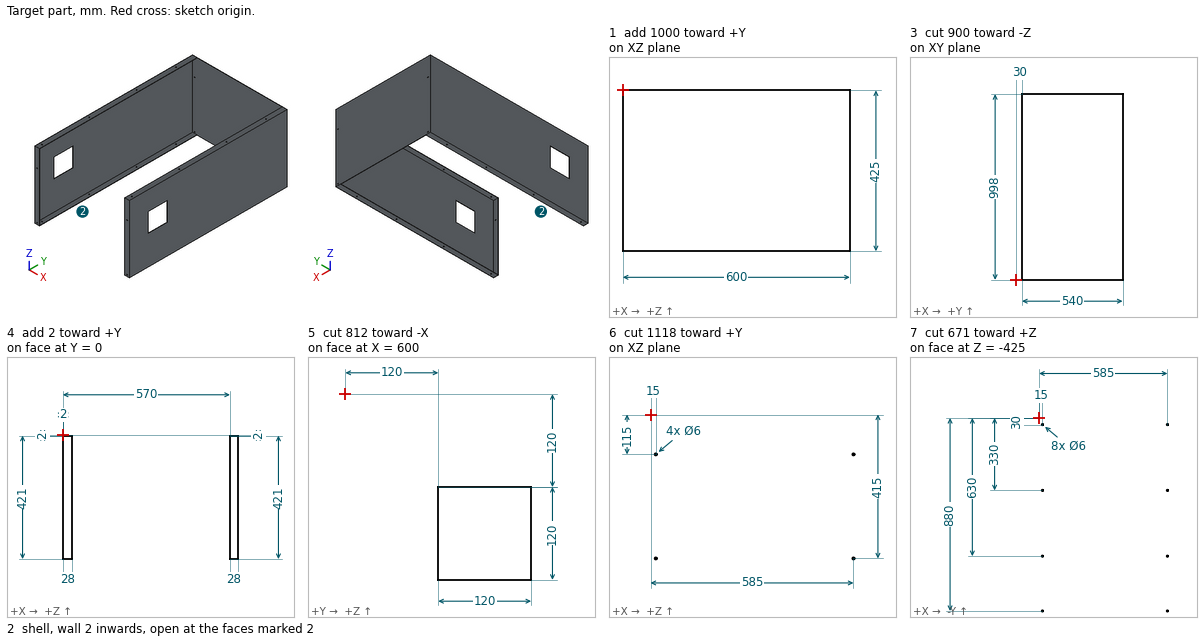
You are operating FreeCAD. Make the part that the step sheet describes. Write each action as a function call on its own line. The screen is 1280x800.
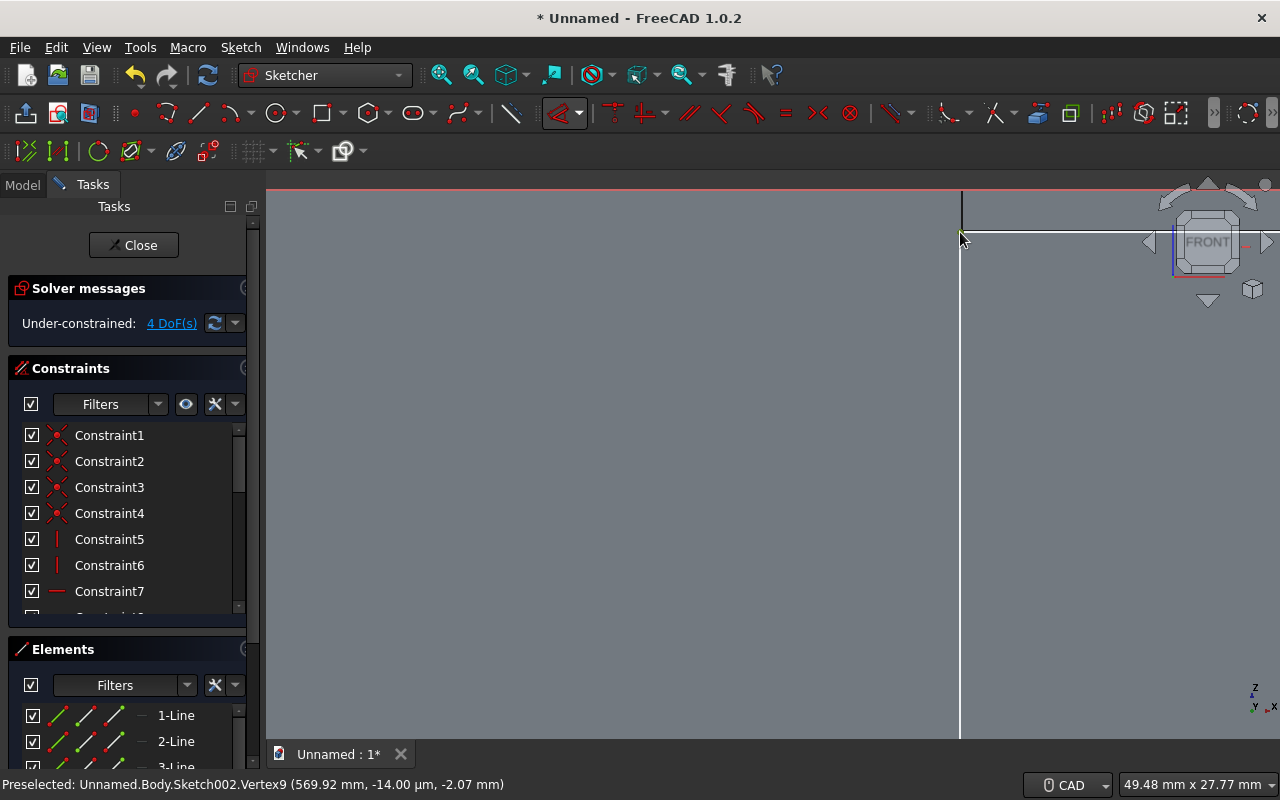
key(i)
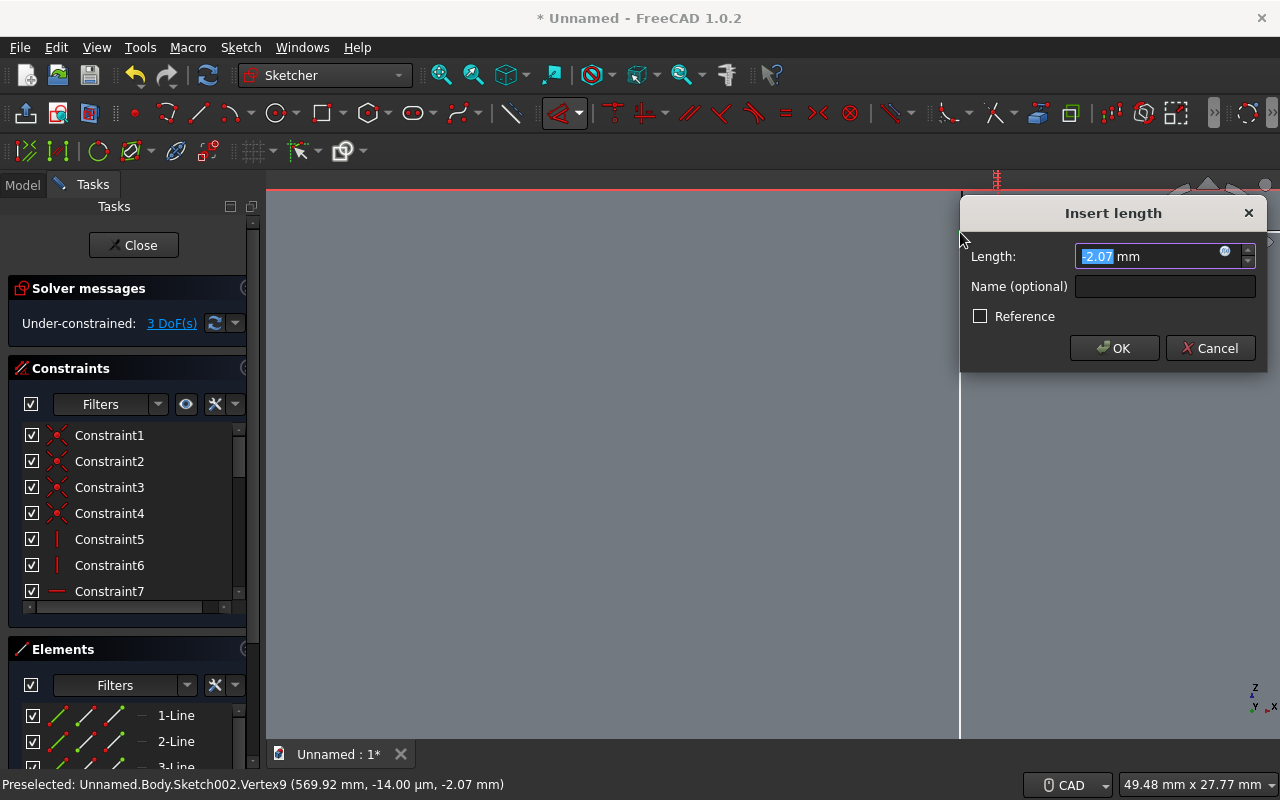
text(-2)
key(Return)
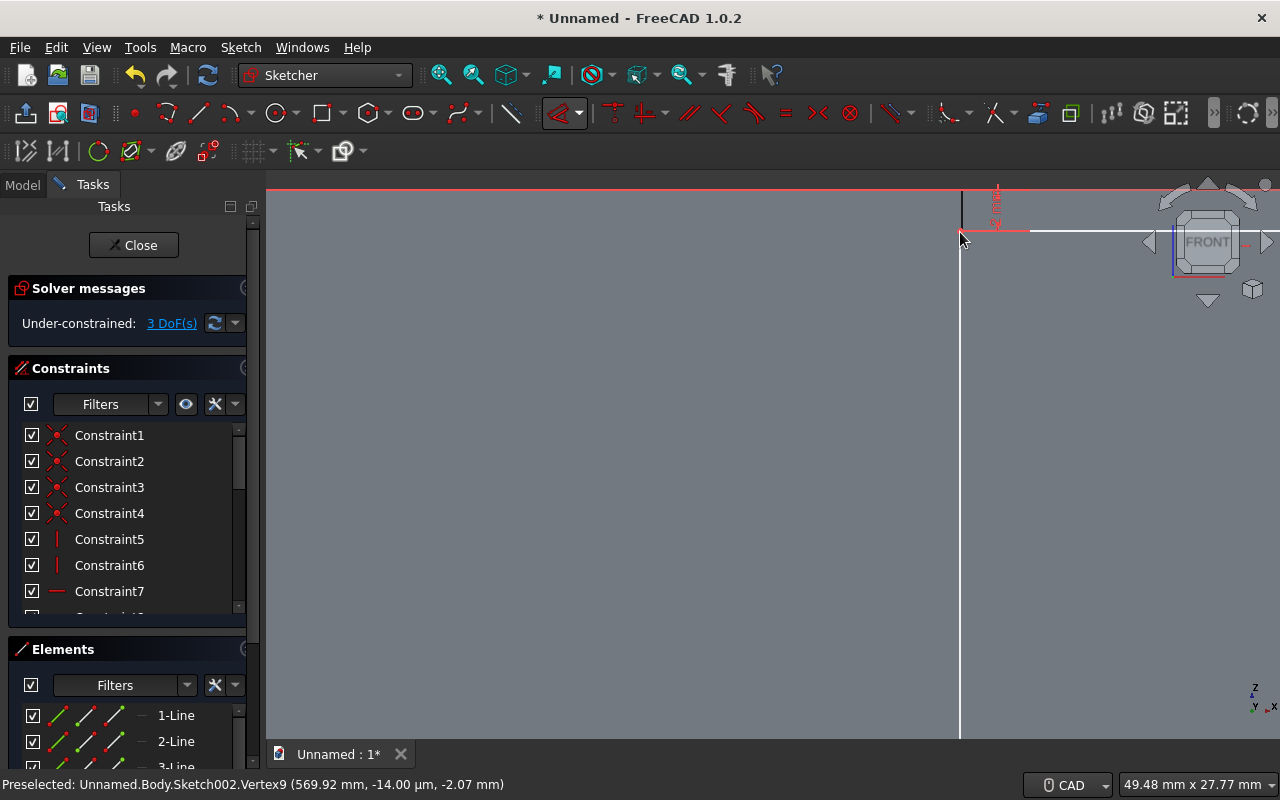
scroll(982, 241, down, 15)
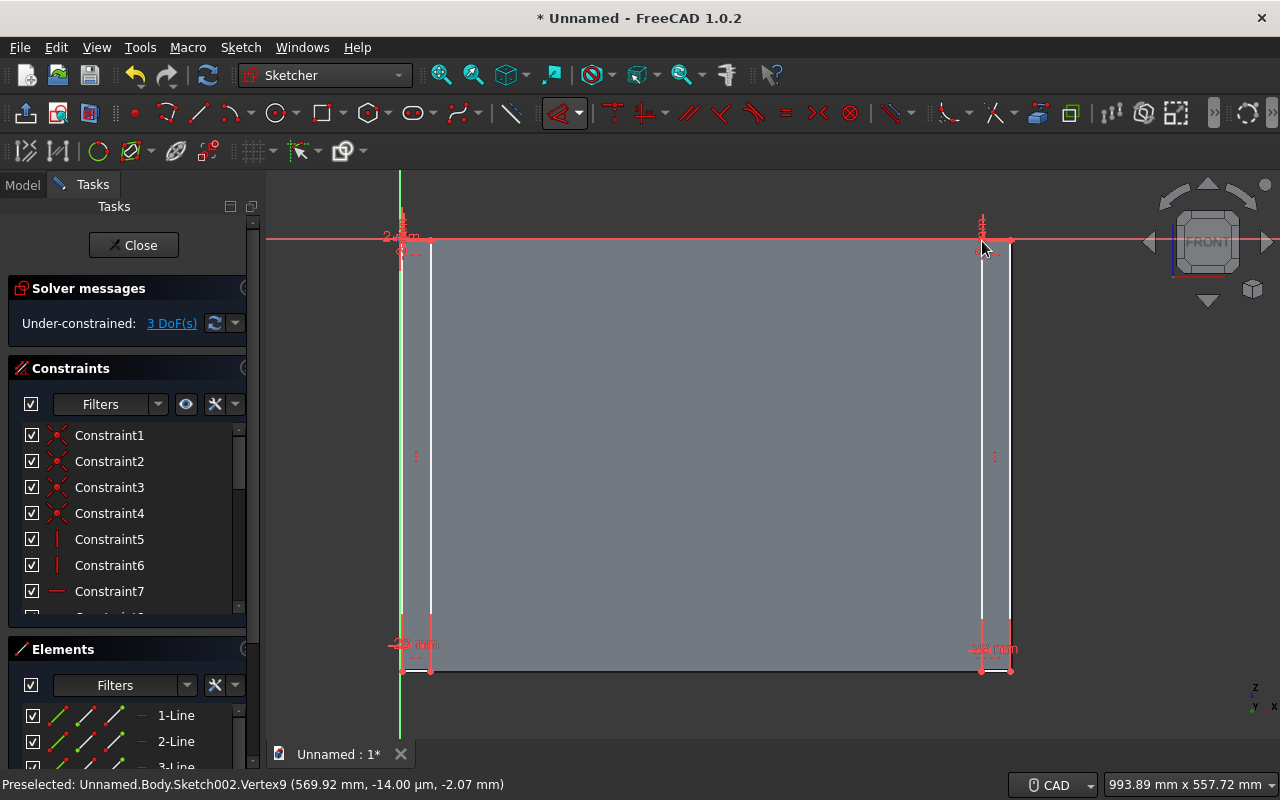
scroll(402, 370, up, 10)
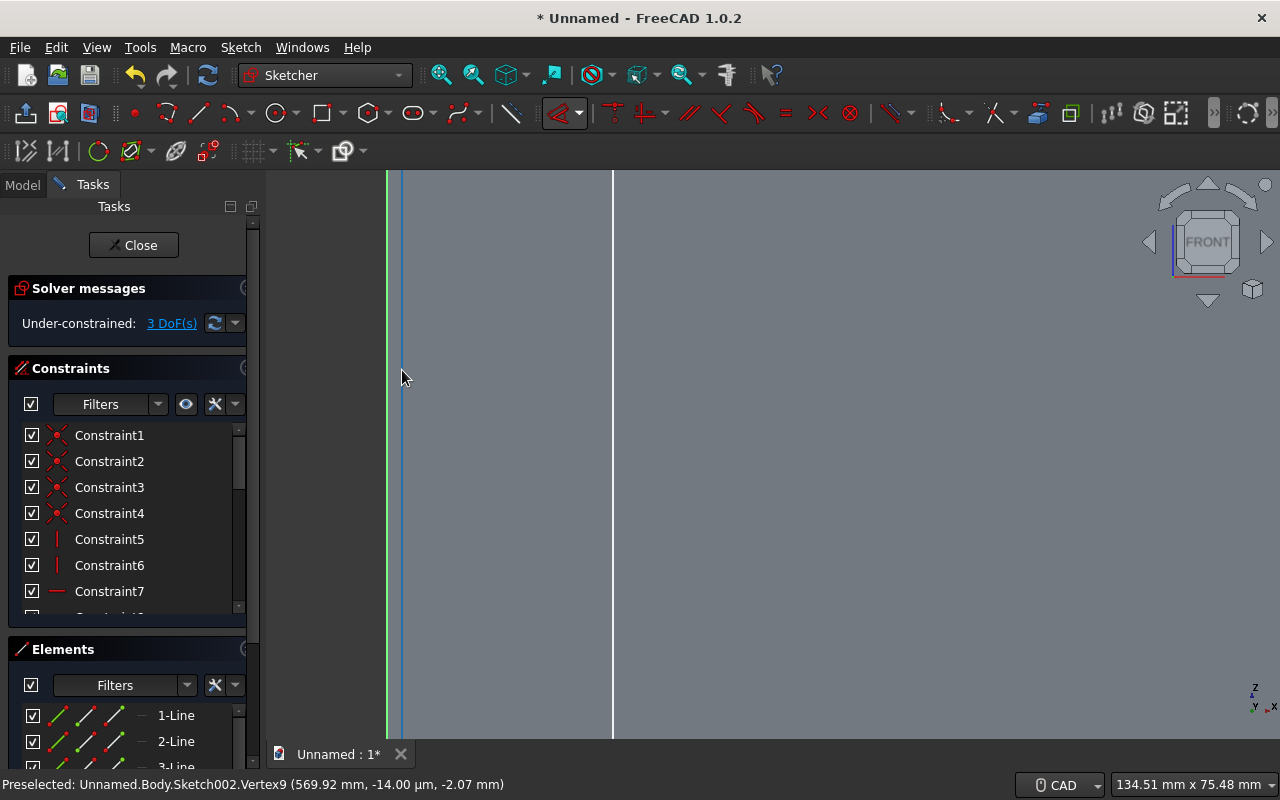
click(402, 367)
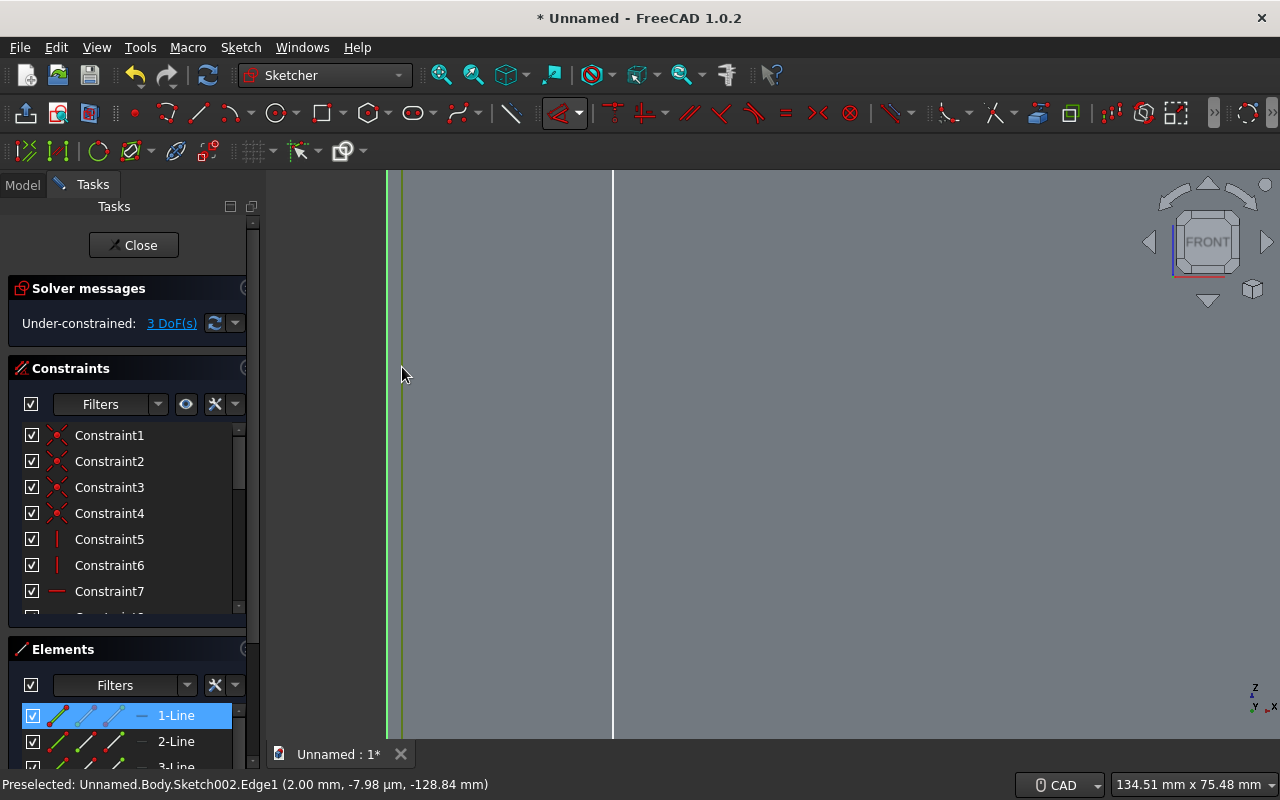
click(582, 114)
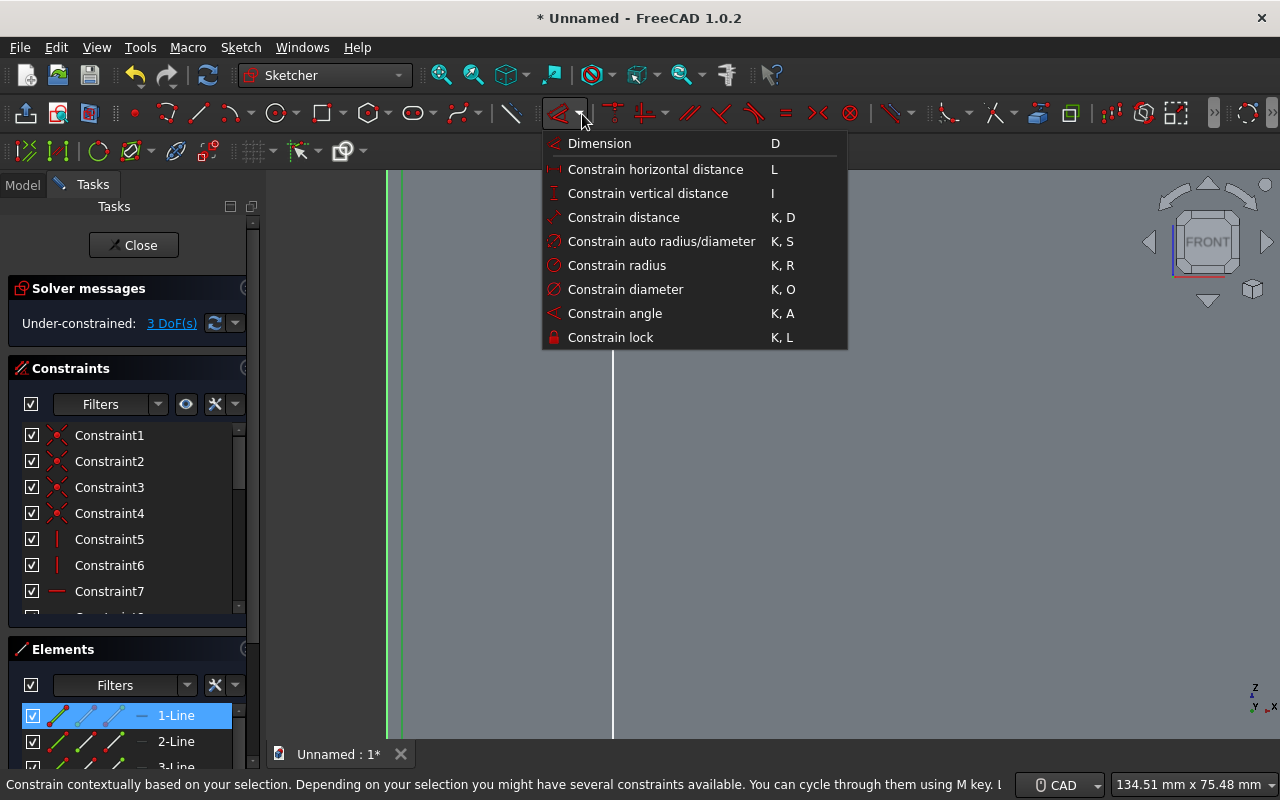
click(695, 193)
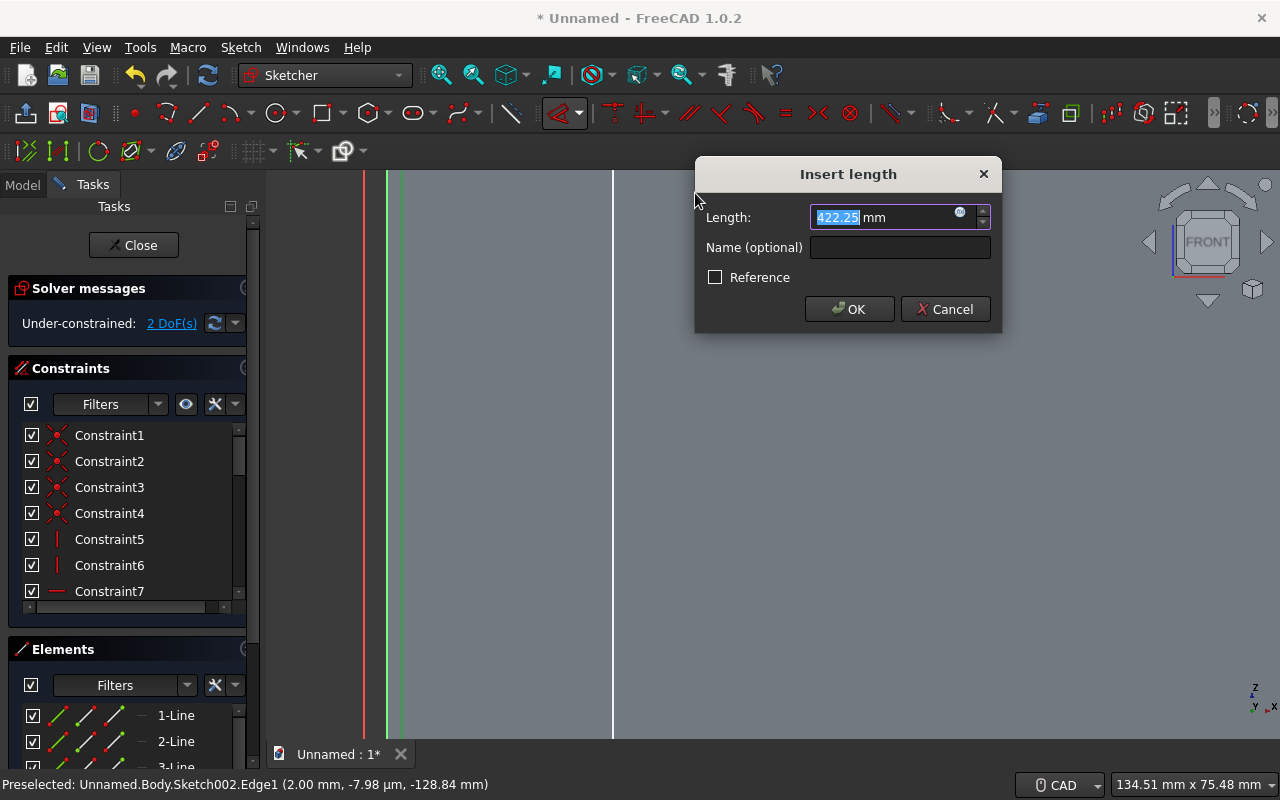
text(421)
key(Return)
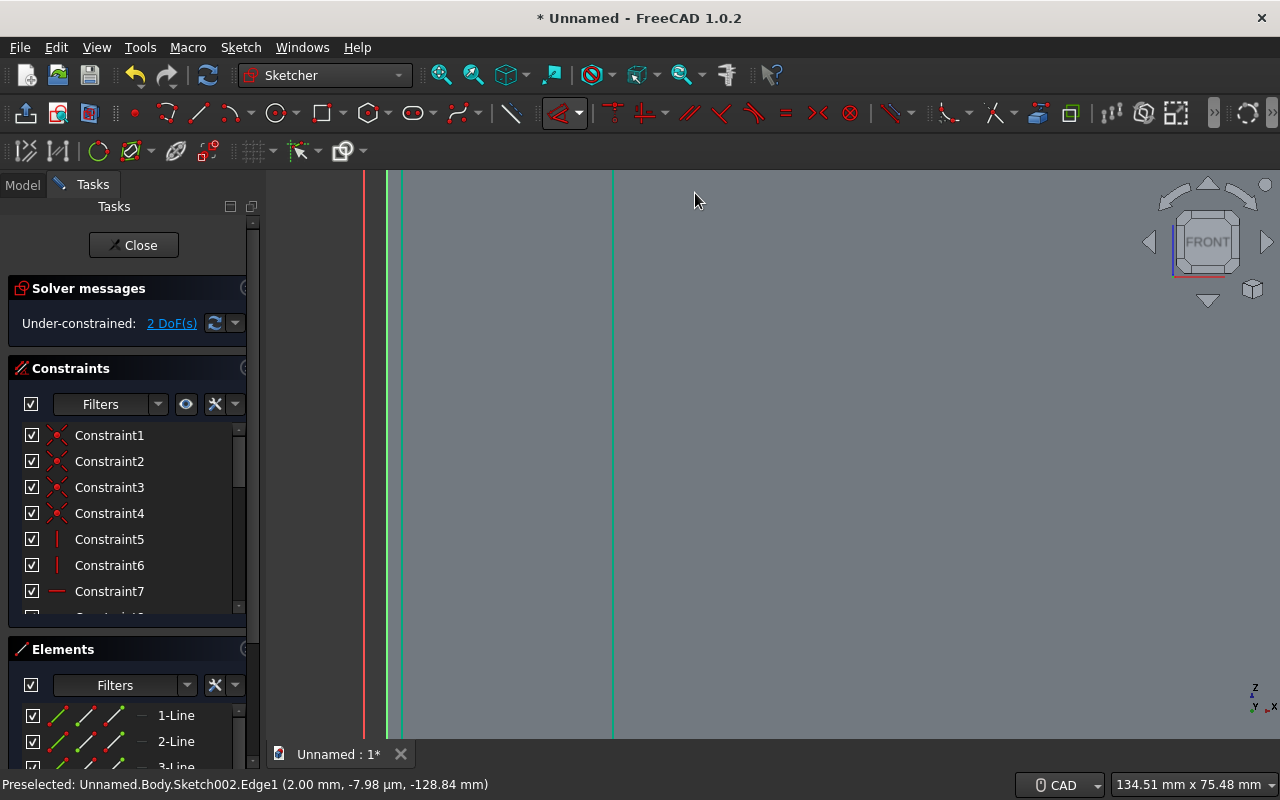
scroll(463, 388, down, 11)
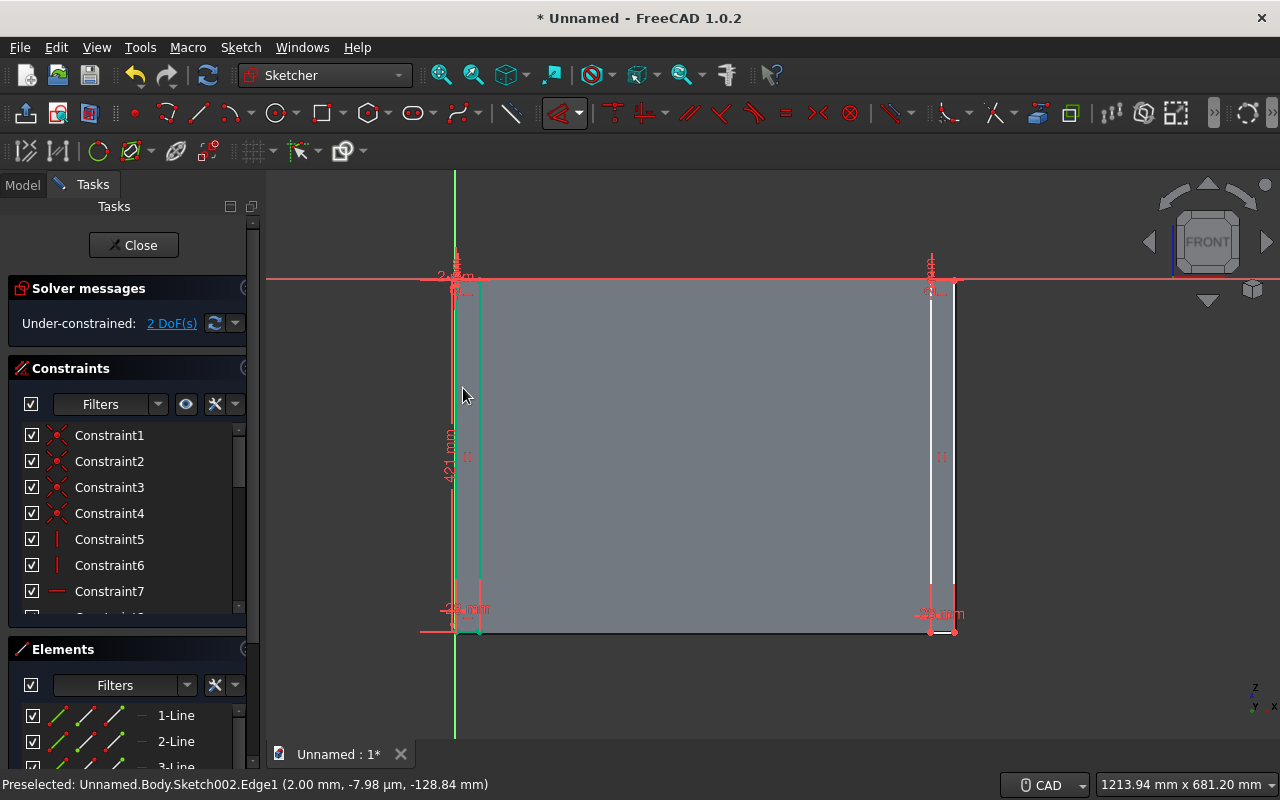
click(931, 386)